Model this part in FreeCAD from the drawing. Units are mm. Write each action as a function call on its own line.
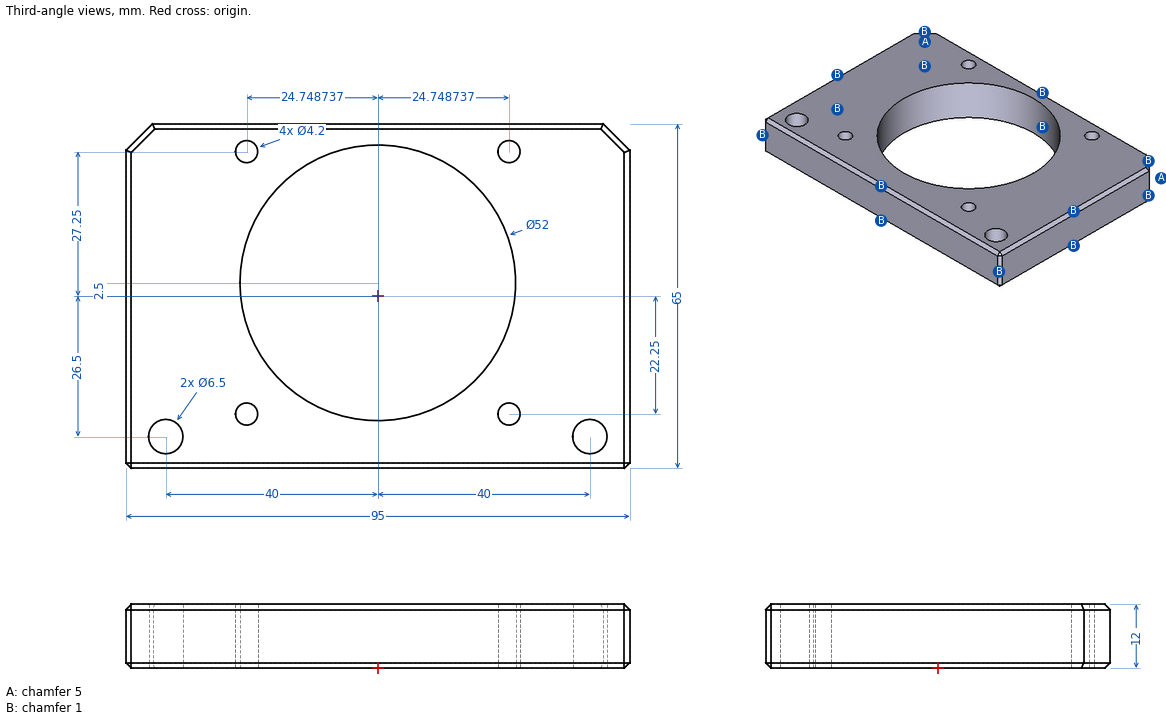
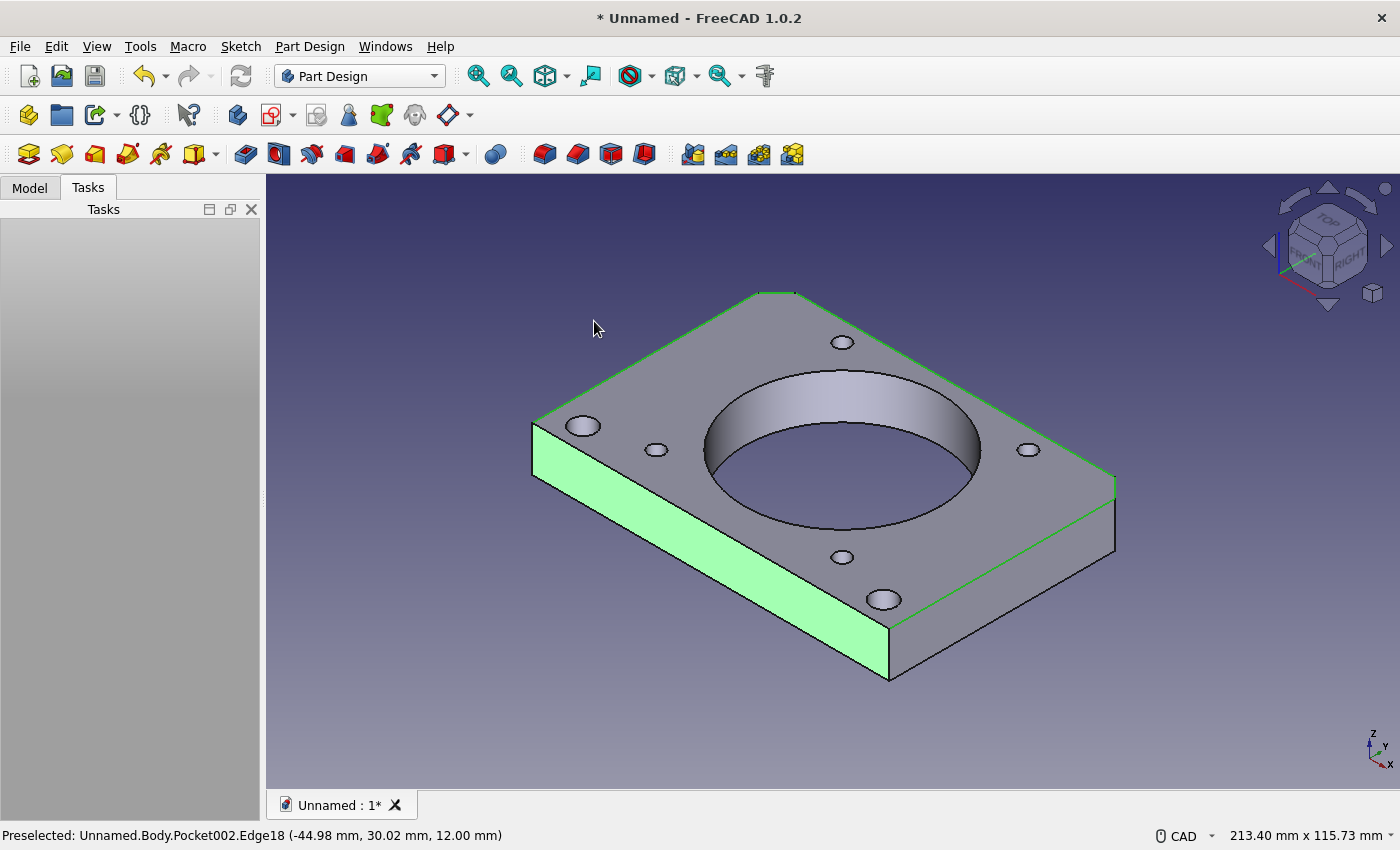
key(1)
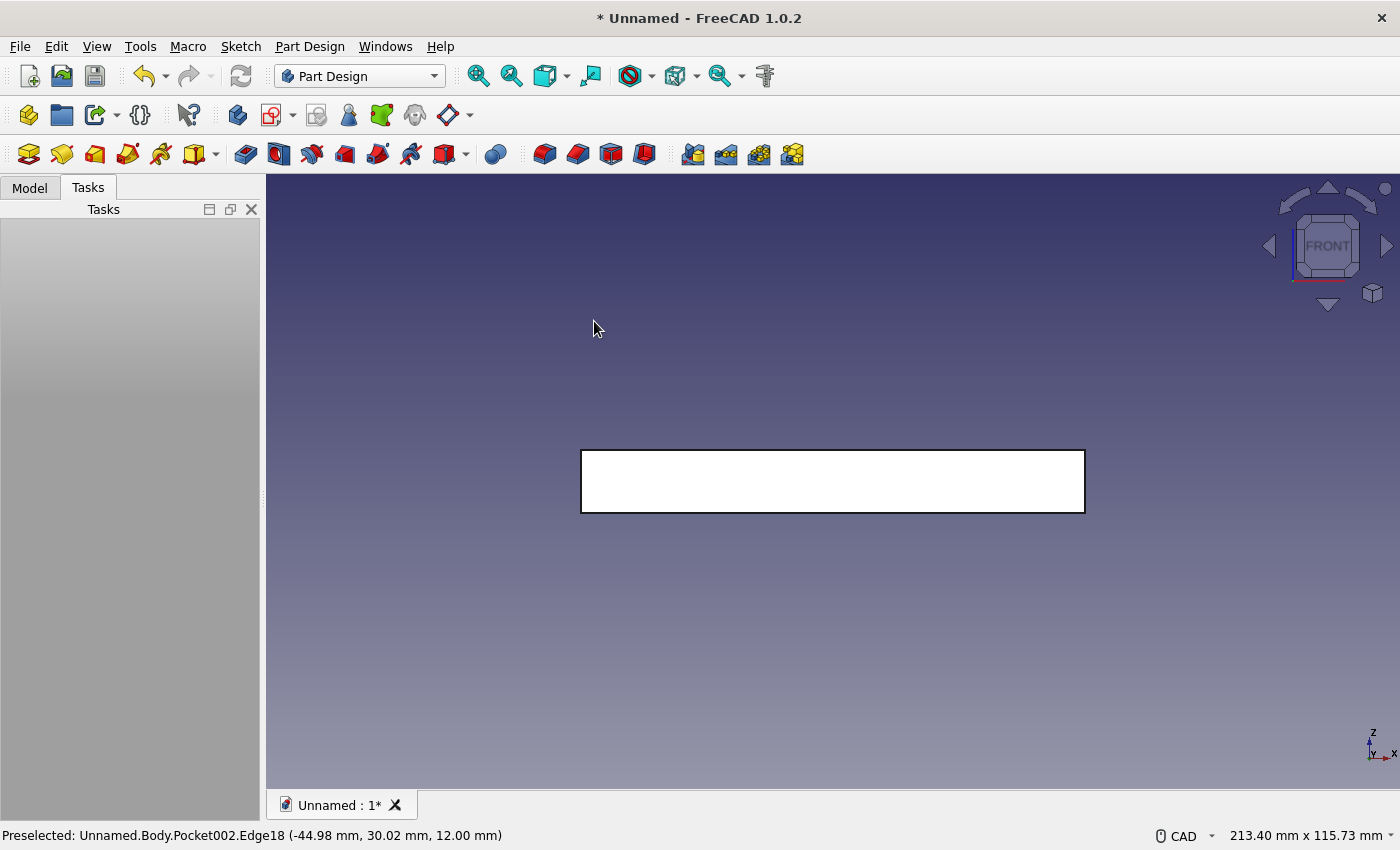
click(479, 76)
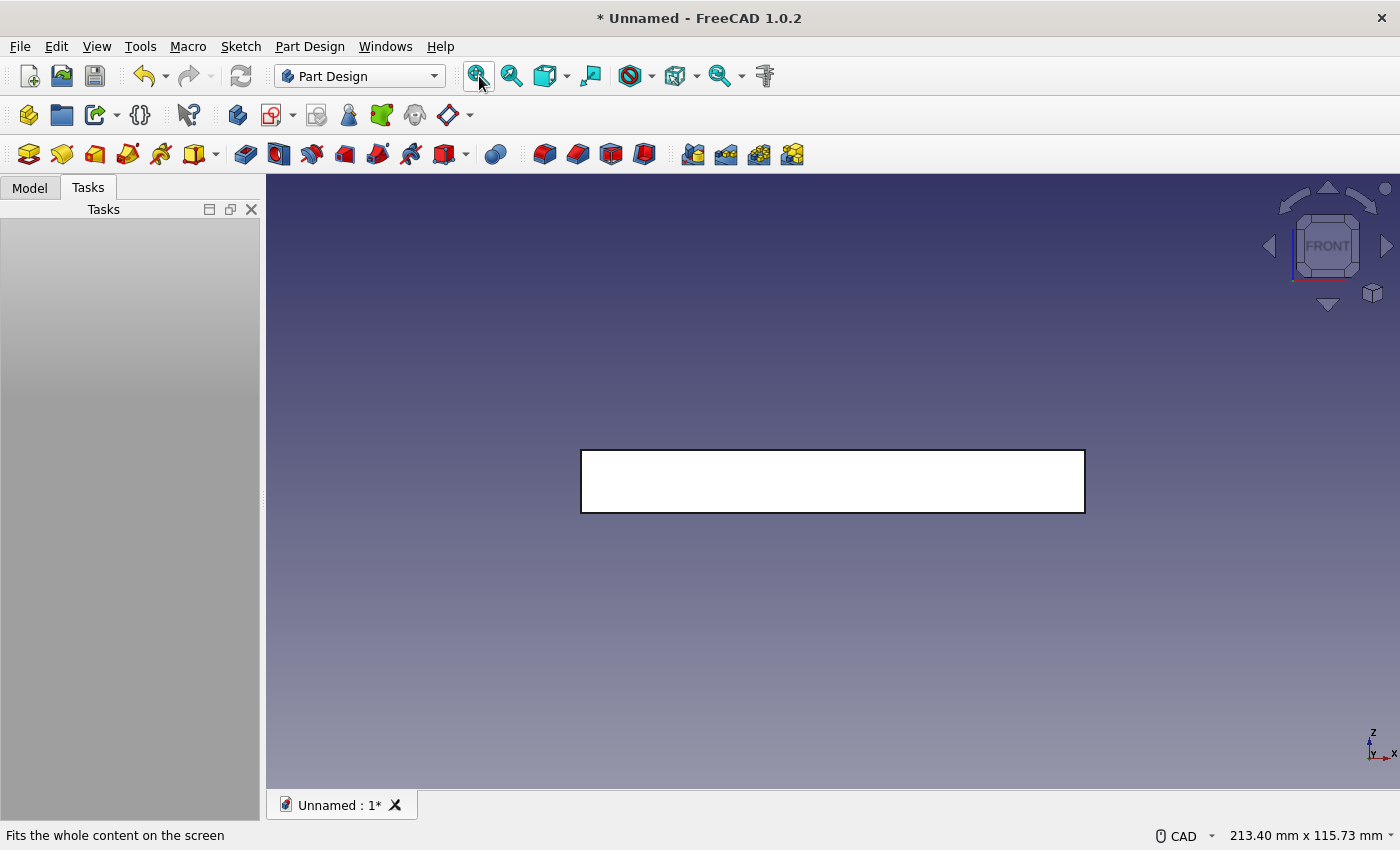
key(3)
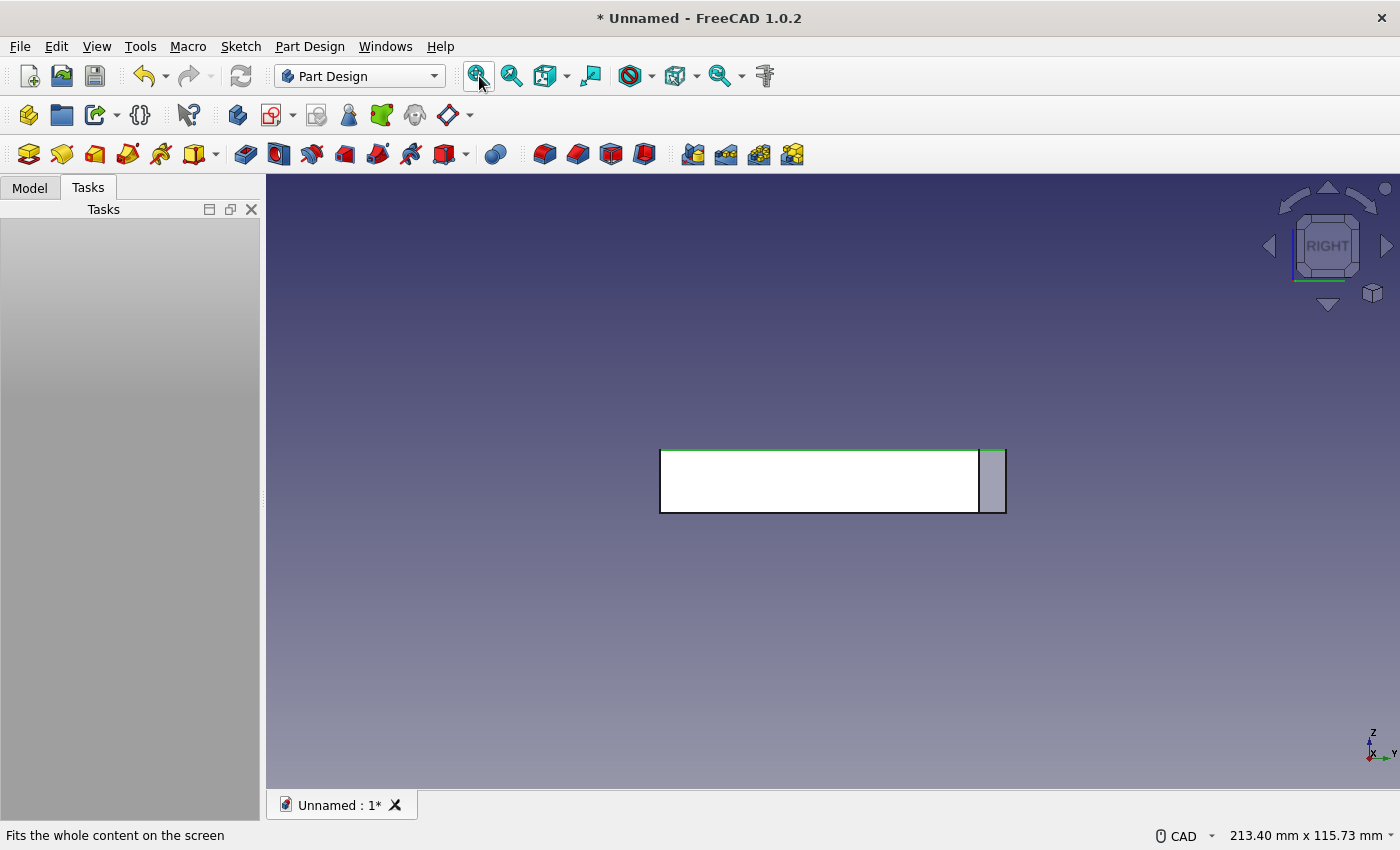
click(479, 76)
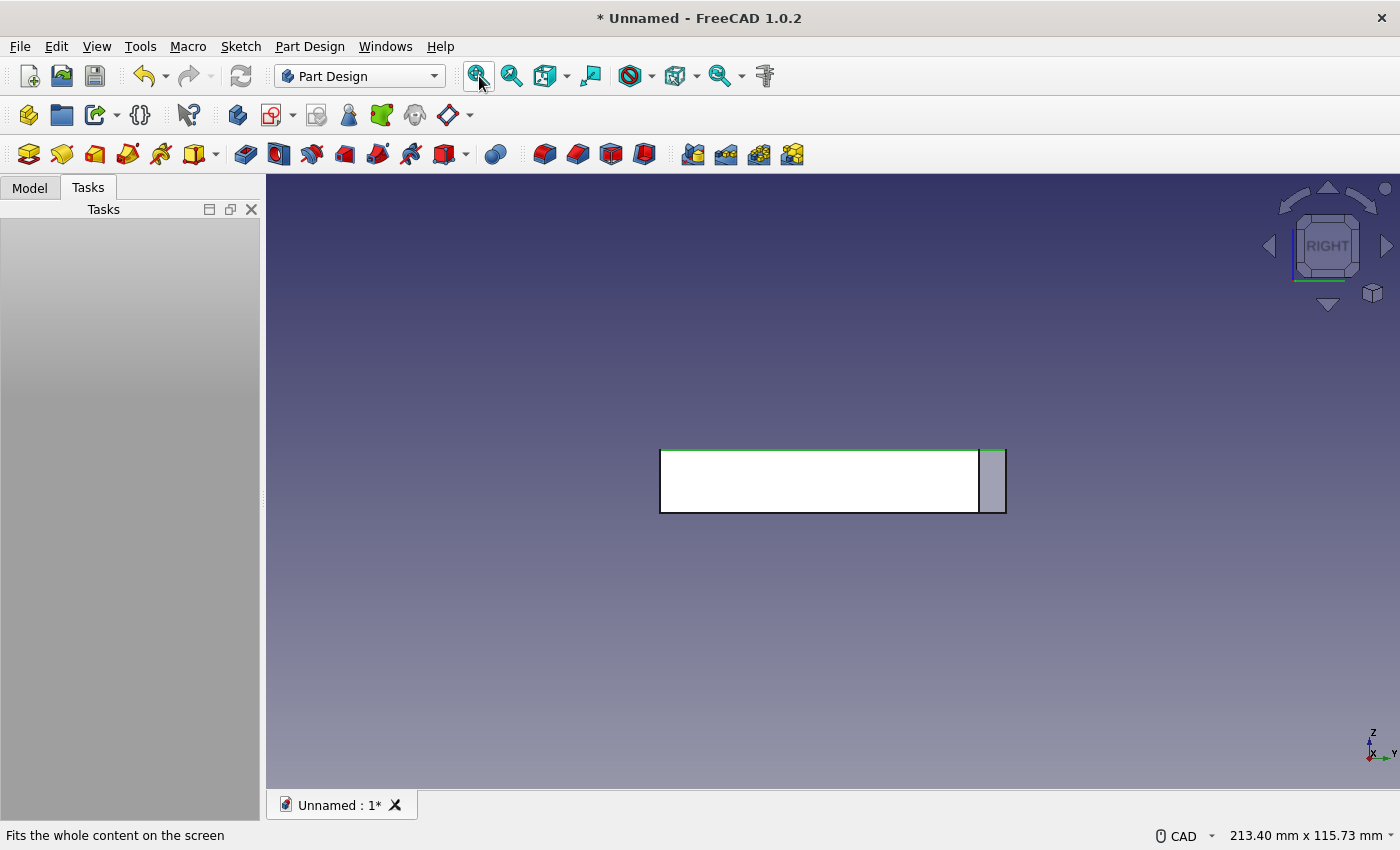
click(992, 512, ctrl)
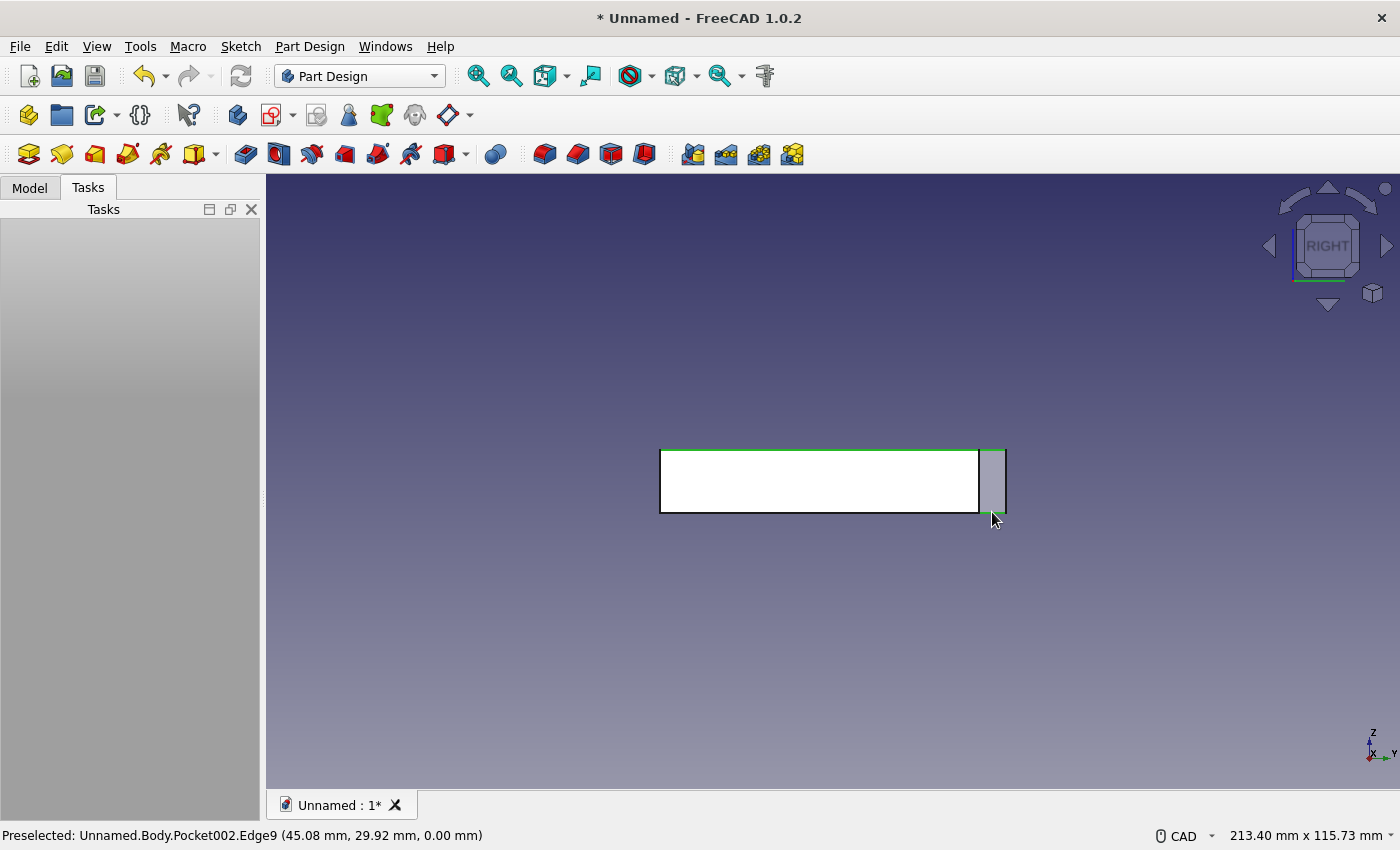
click(820, 512, ctrl)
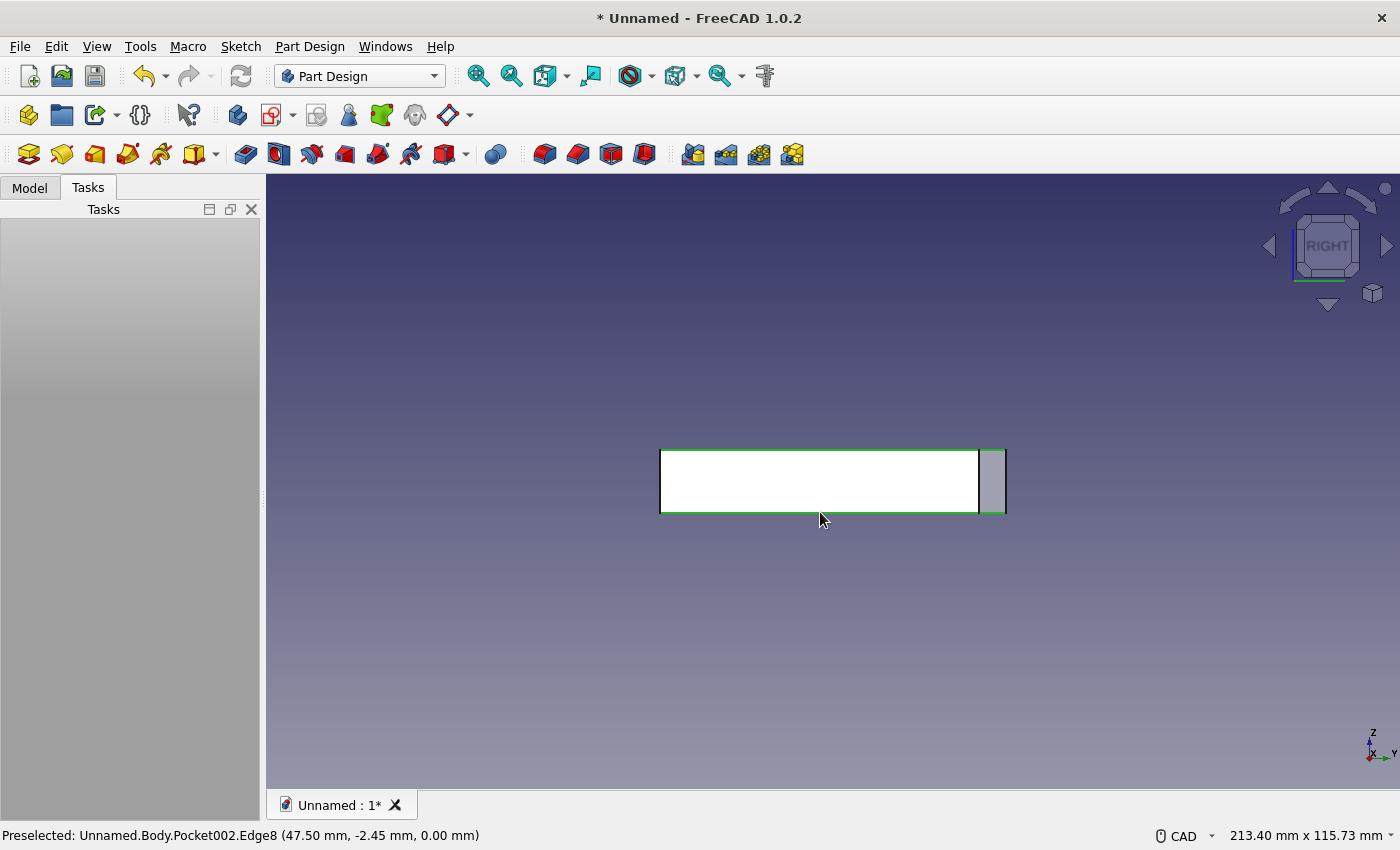
key(5)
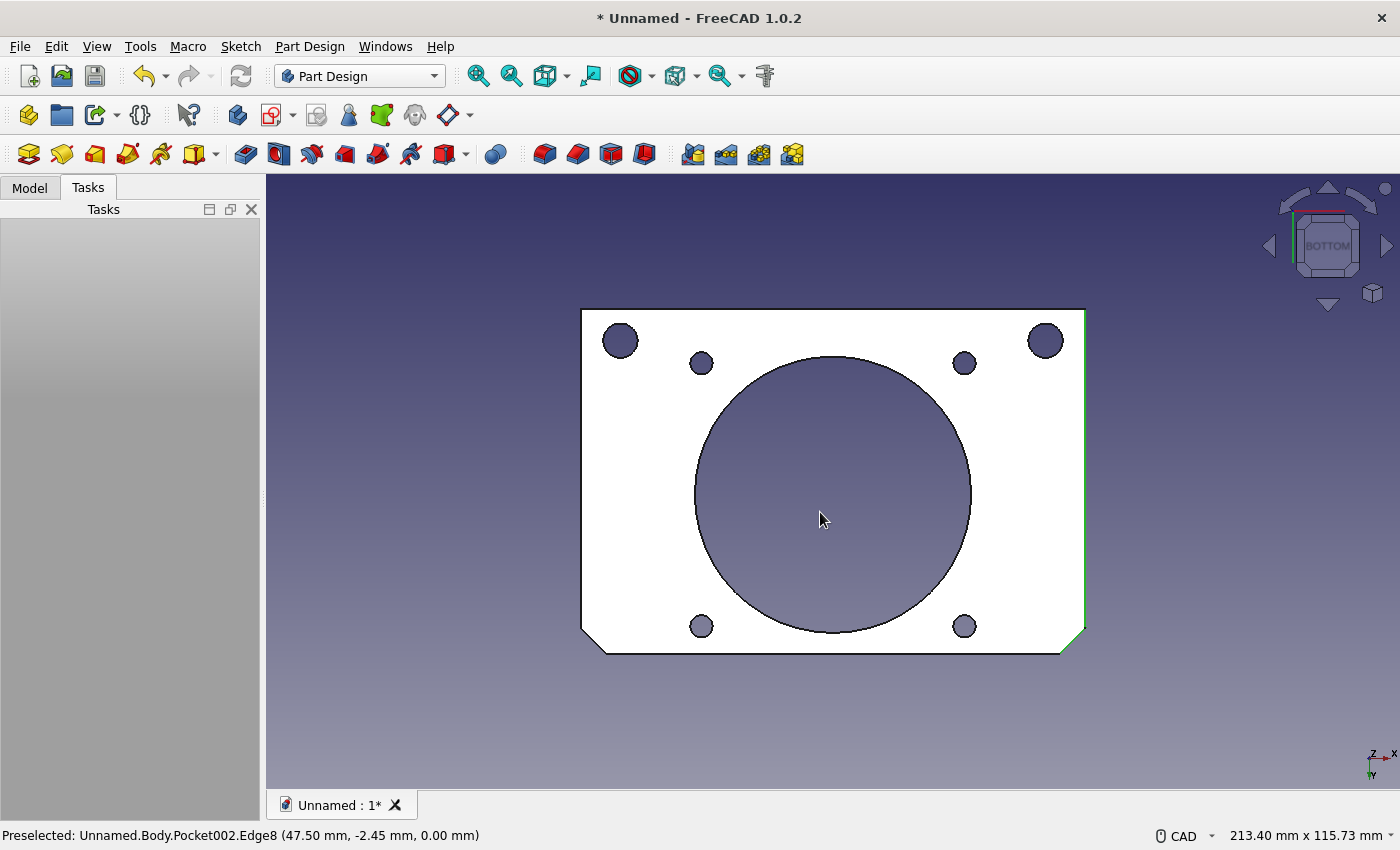
click(833, 653, ctrl)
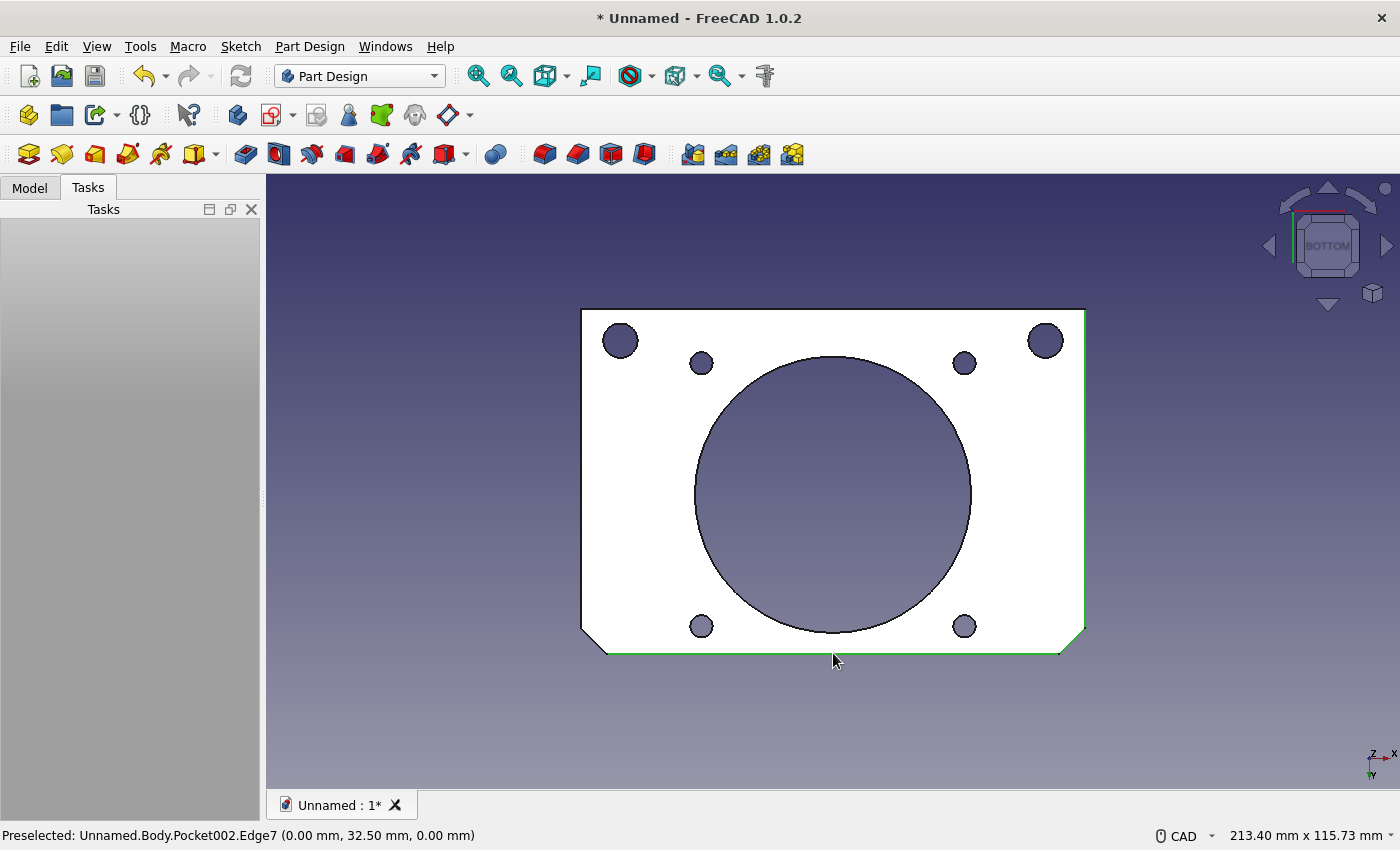
click(581, 467, ctrl)